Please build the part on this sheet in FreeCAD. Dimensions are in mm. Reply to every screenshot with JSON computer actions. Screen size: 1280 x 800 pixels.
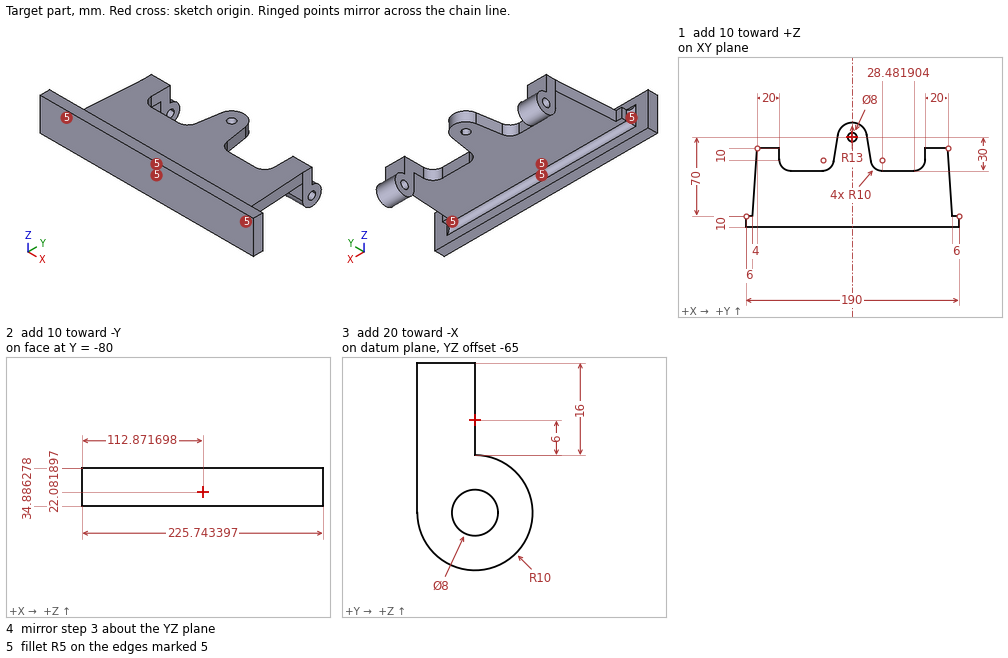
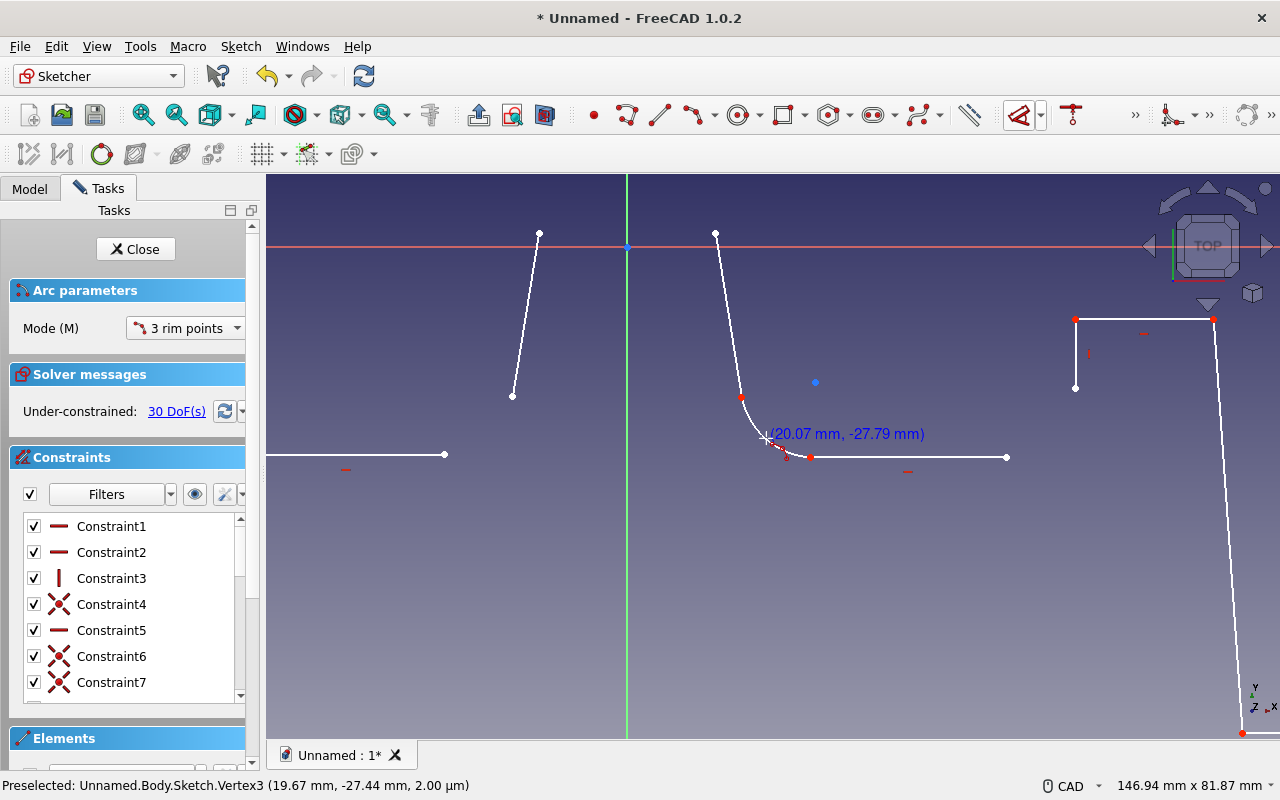
{"action": "left_click", "coordinate": [716, 234]}
{"action": "left_click", "coordinate": [539, 234]}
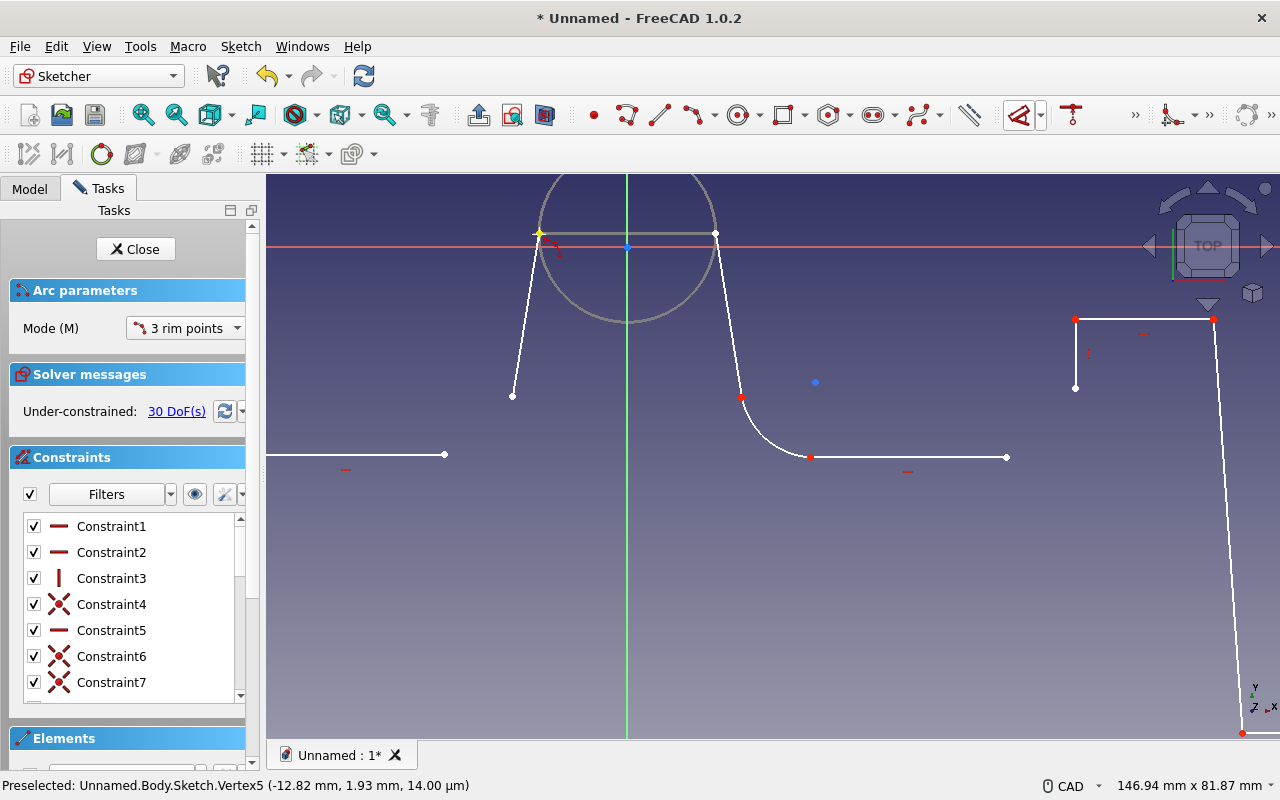
{"action": "scroll", "coordinate": [767, 439], "scroll_direction": "down", "scroll_amount": 4}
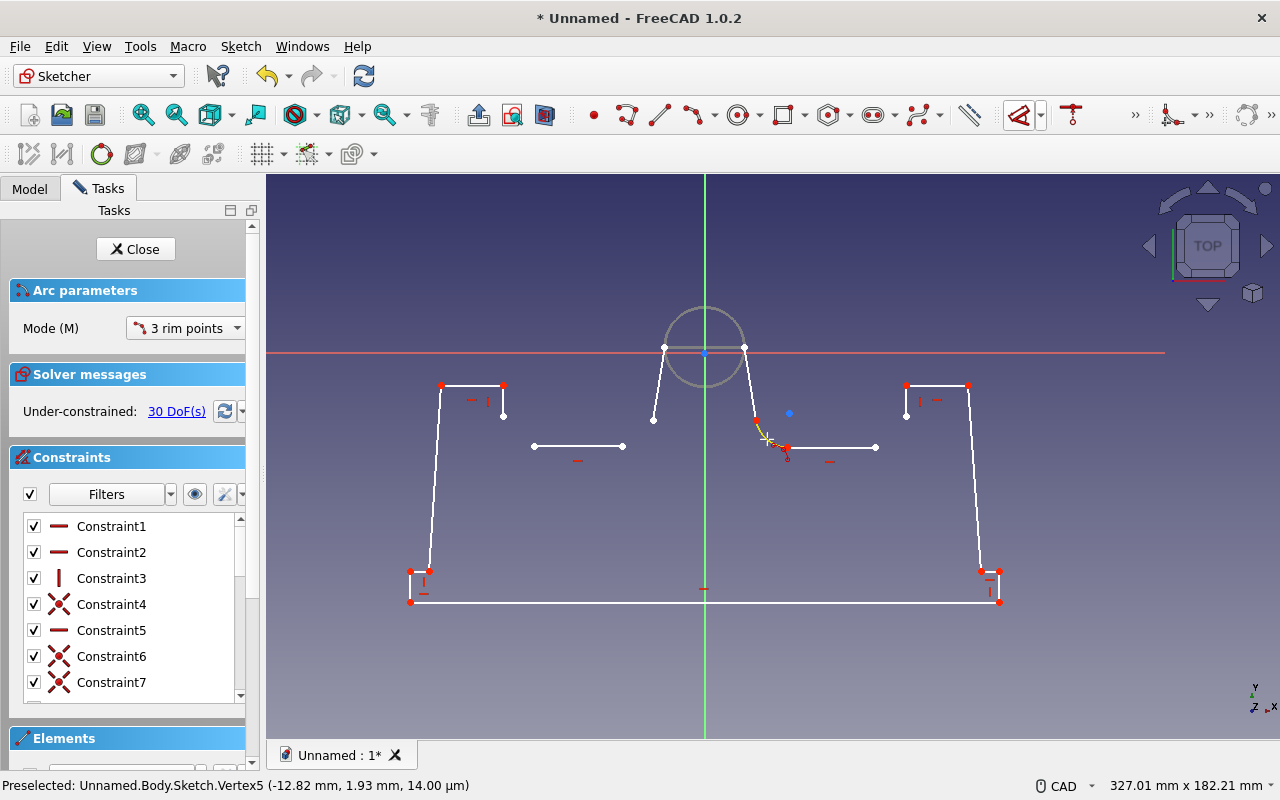
{"action": "left_click", "coordinate": [726, 319]}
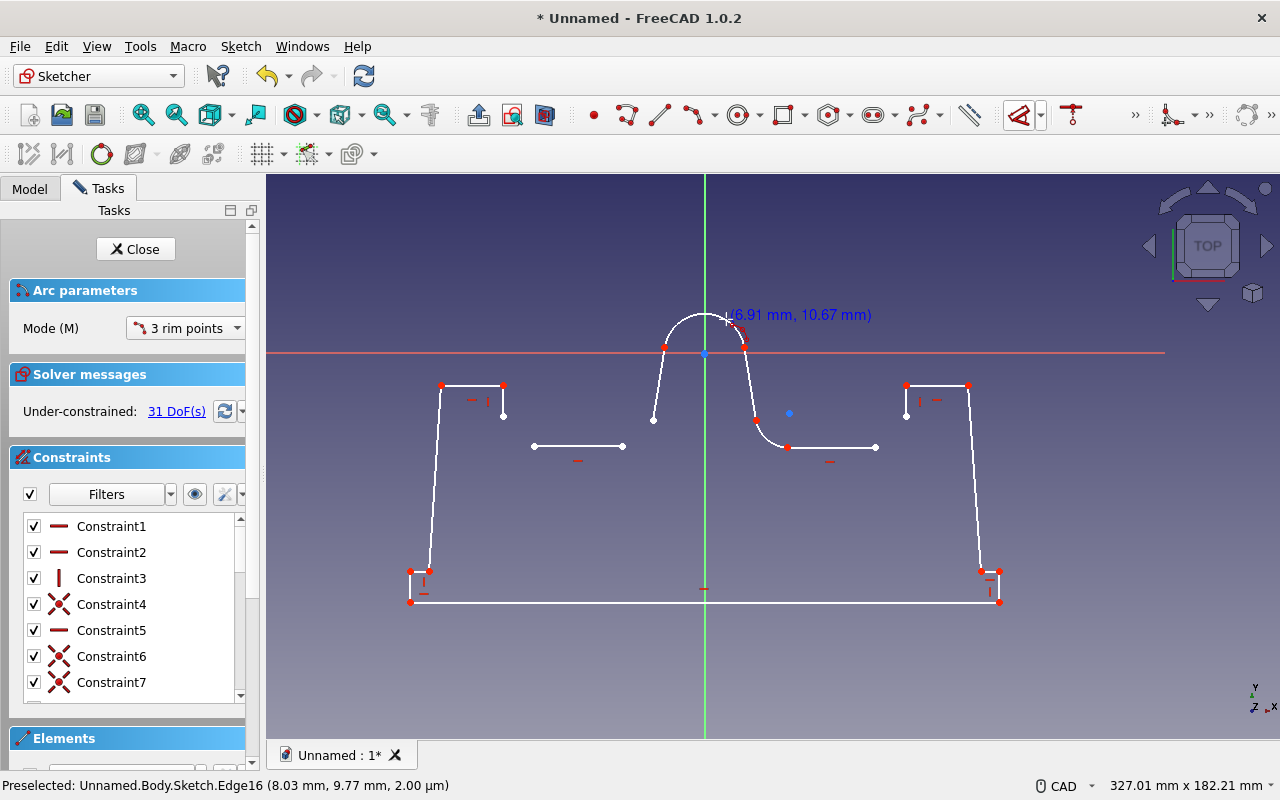
{"action": "left_click", "coordinate": [653, 420]}
{"action": "left_click", "coordinate": [623, 446]}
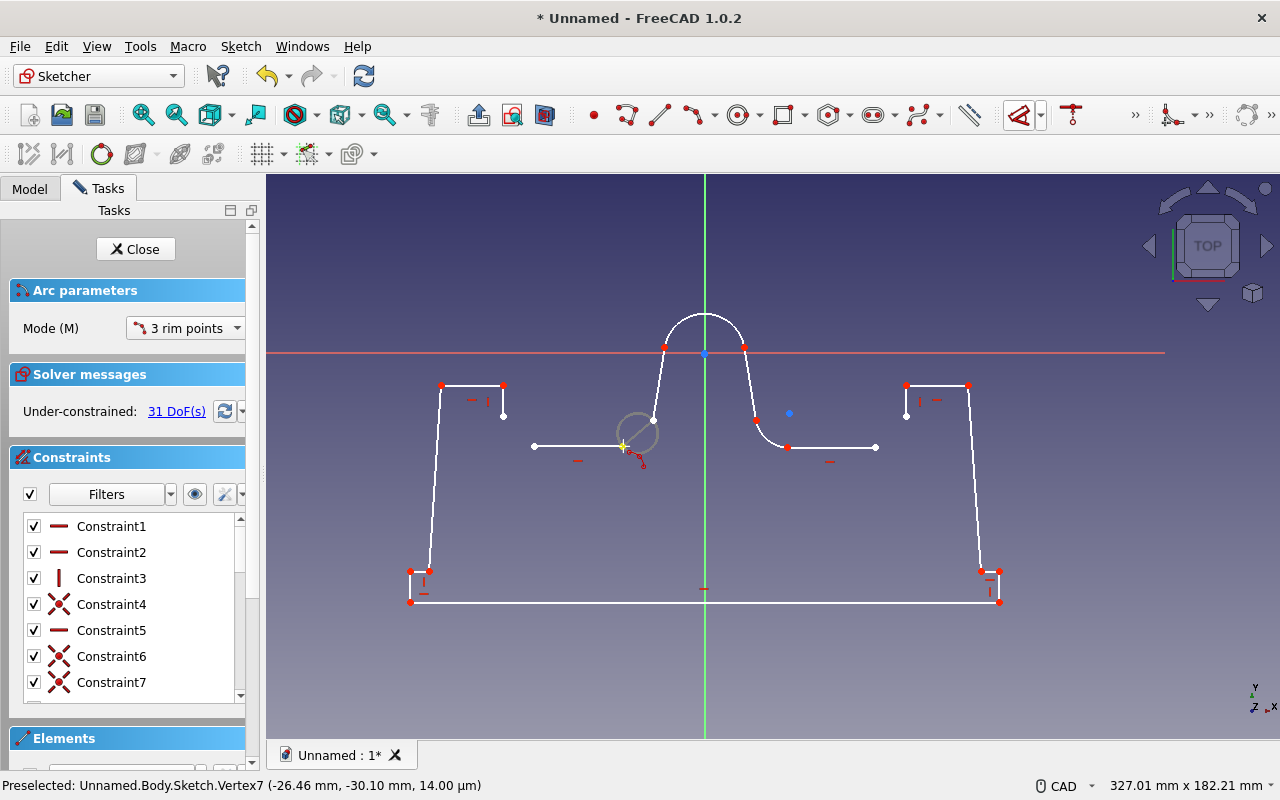
{"action": "scroll", "coordinate": [642, 439], "scroll_direction": "up", "scroll_amount": 4}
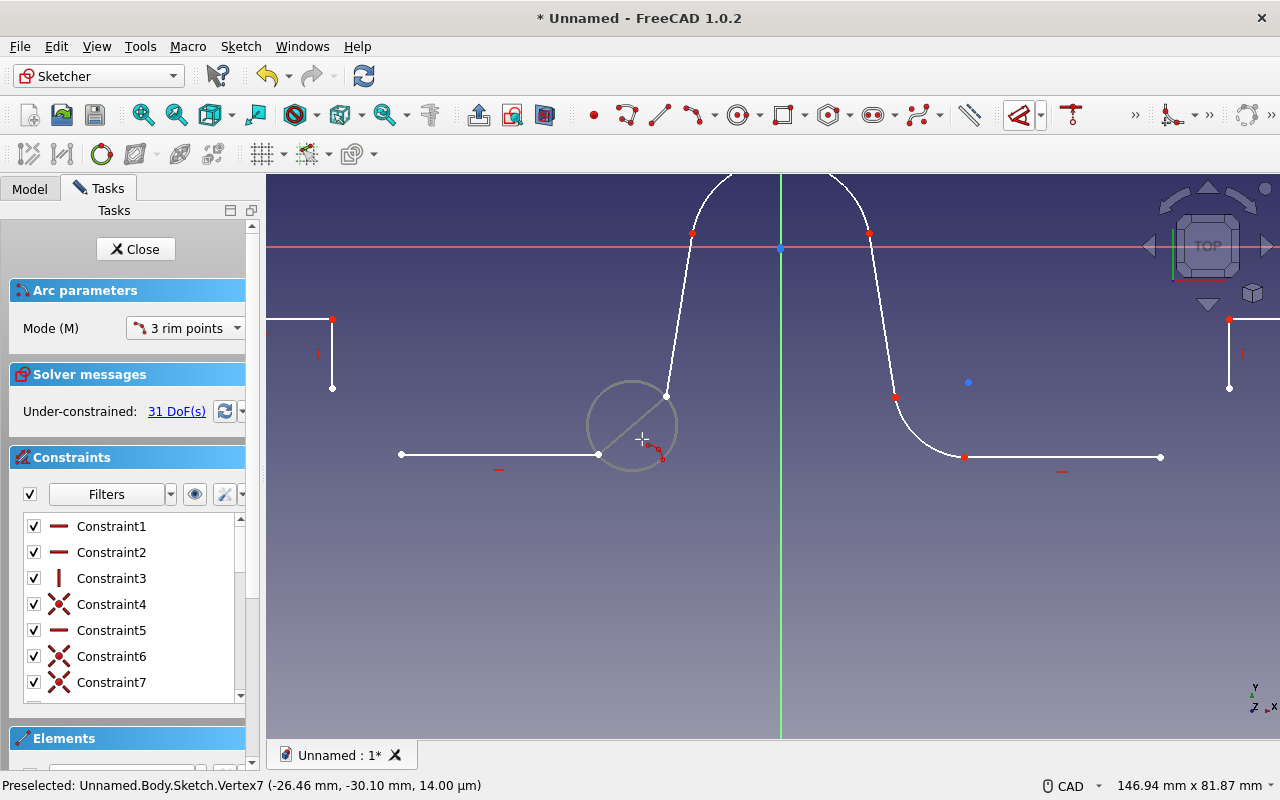
{"action": "left_click", "coordinate": [643, 438]}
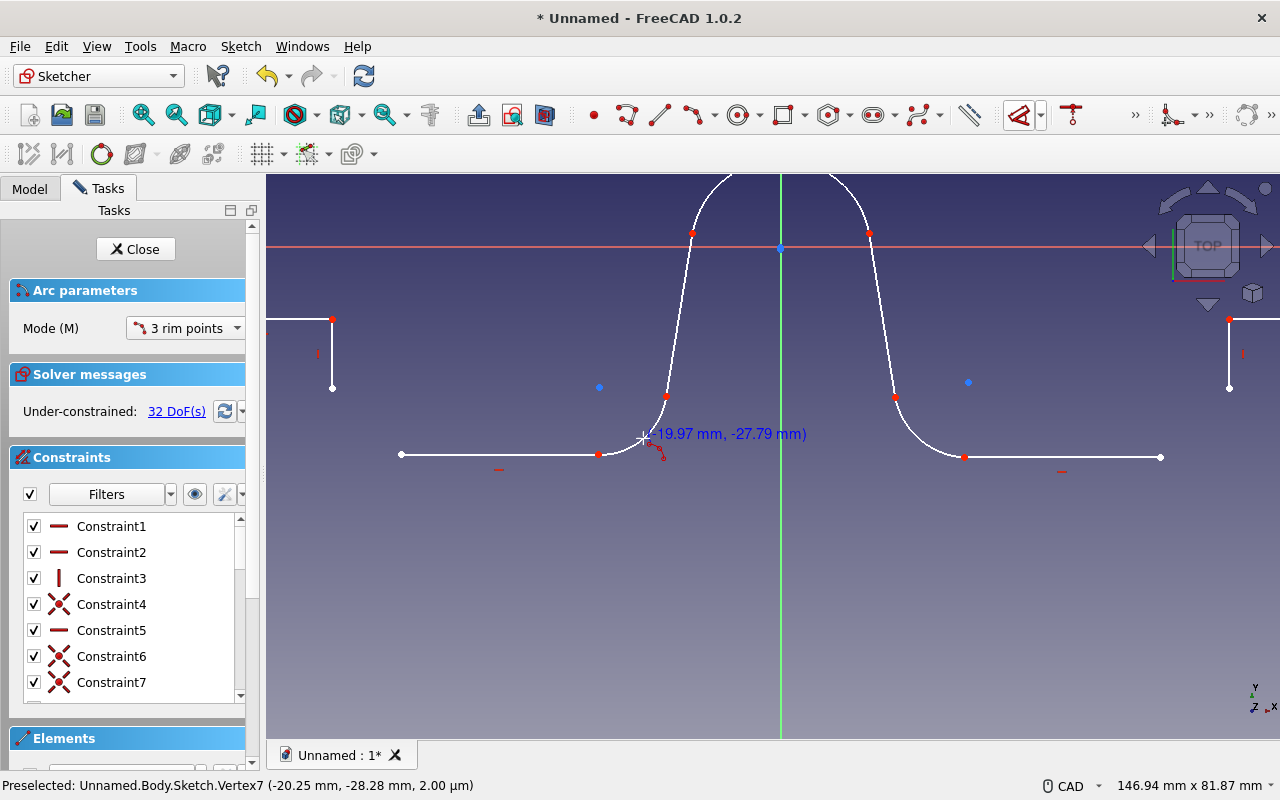
{"action": "left_click", "coordinate": [401, 455]}
{"action": "left_click", "coordinate": [332, 388]}
{"action": "left_click", "coordinate": [352, 434]}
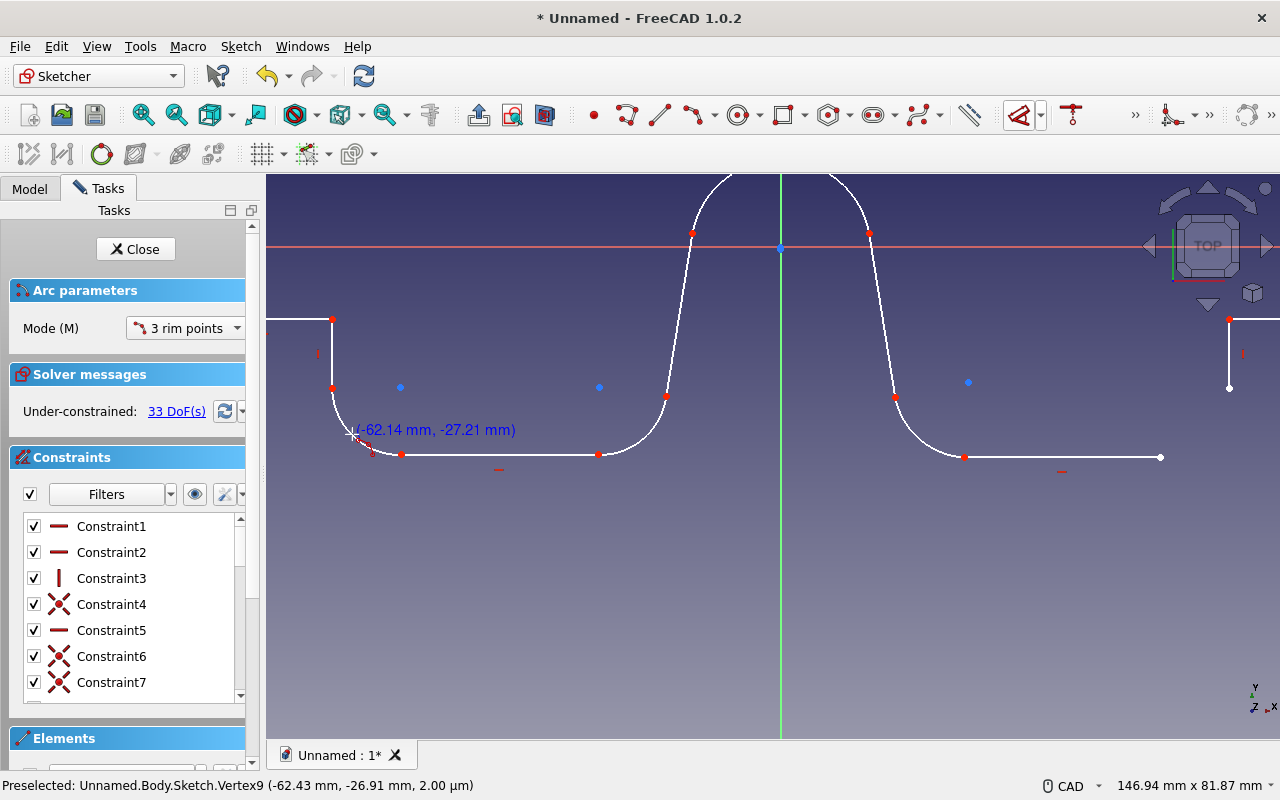
{"action": "scroll", "coordinate": [642, 439], "scroll_direction": "down", "scroll_amount": 4}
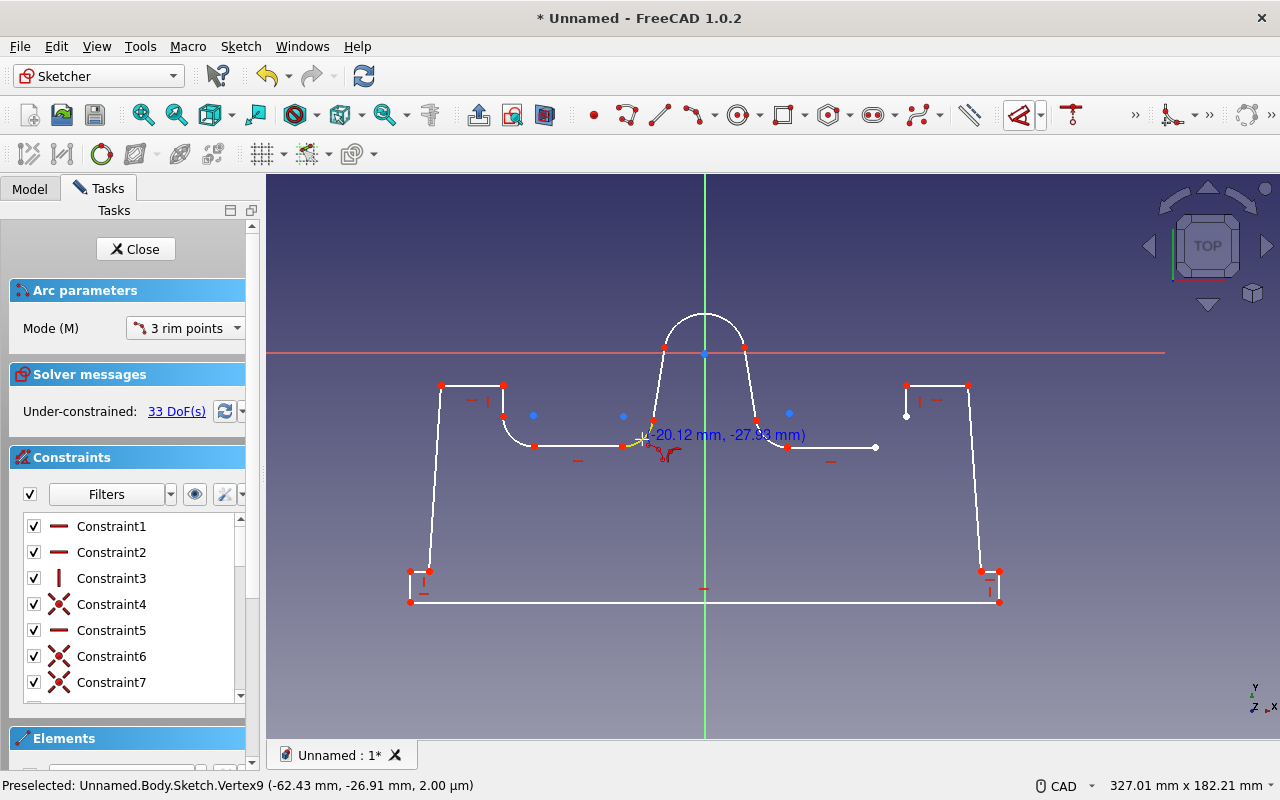
{"action": "left_click", "coordinate": [906, 417]}
{"action": "left_click", "coordinate": [875, 448]}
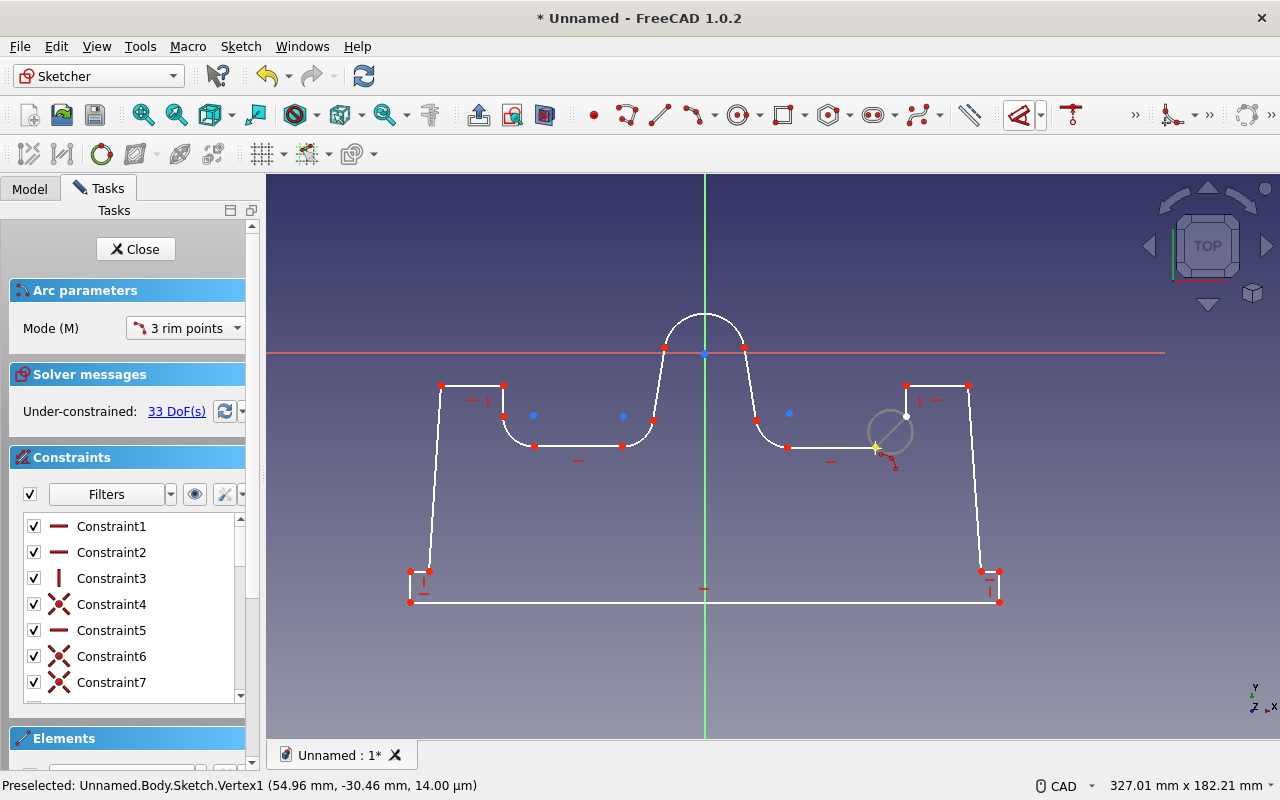
{"action": "scroll", "coordinate": [897, 437], "scroll_direction": "up", "scroll_amount": 3}